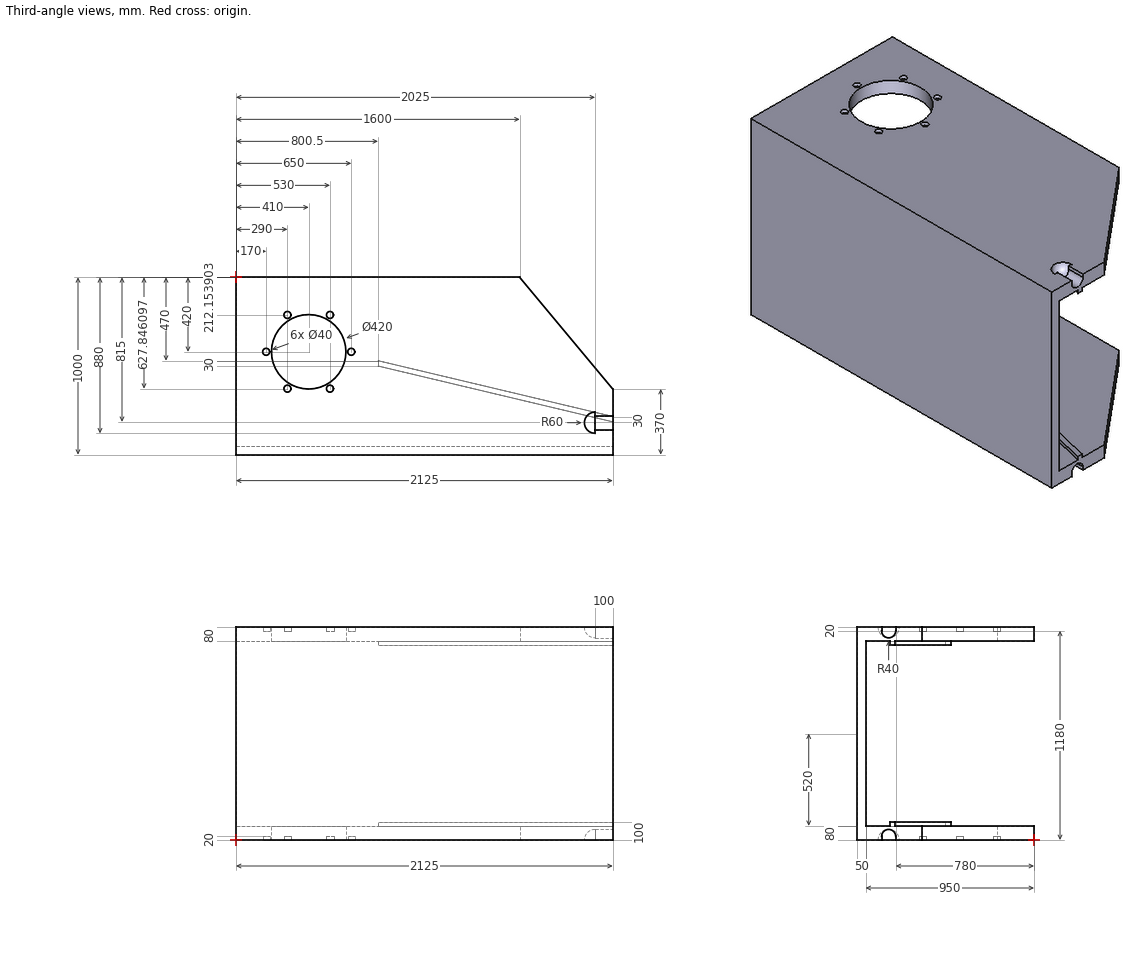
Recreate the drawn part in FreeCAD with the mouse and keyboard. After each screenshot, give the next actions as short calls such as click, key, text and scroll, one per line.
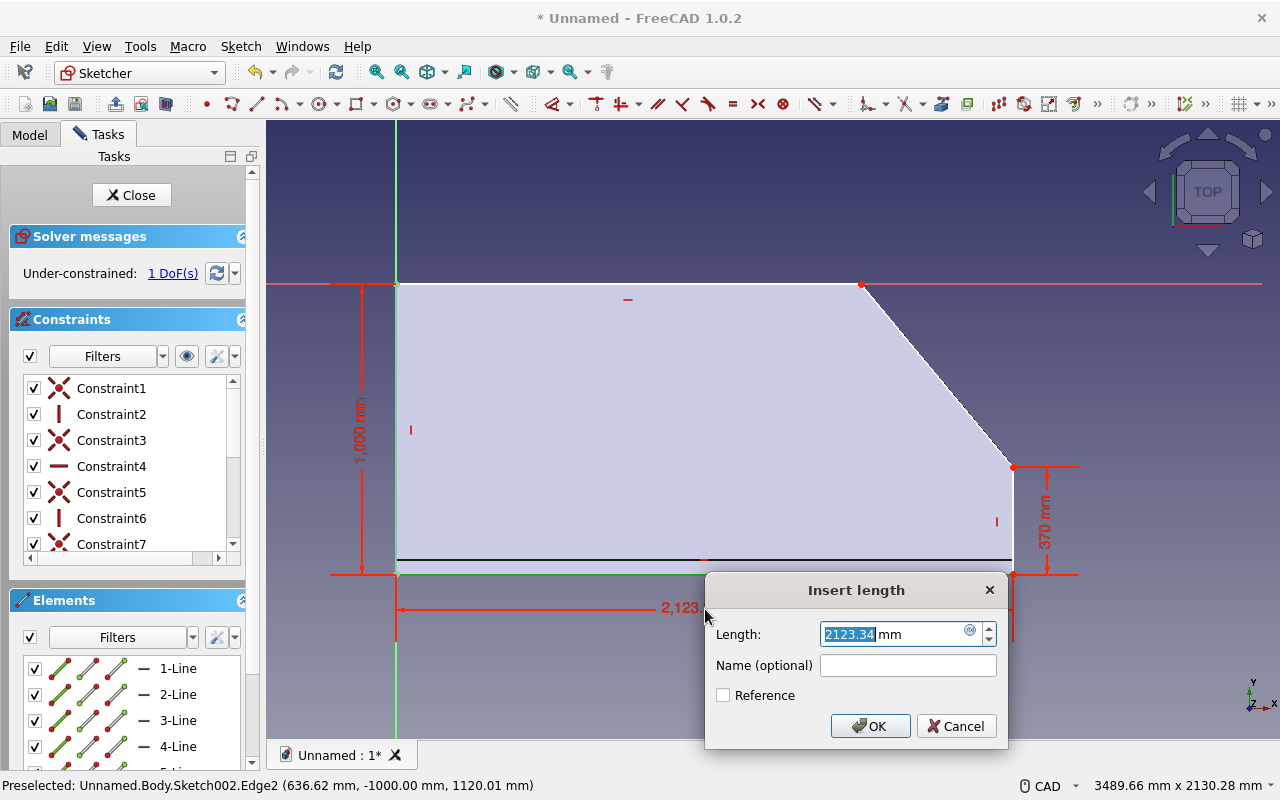
text(2125)
key(Return)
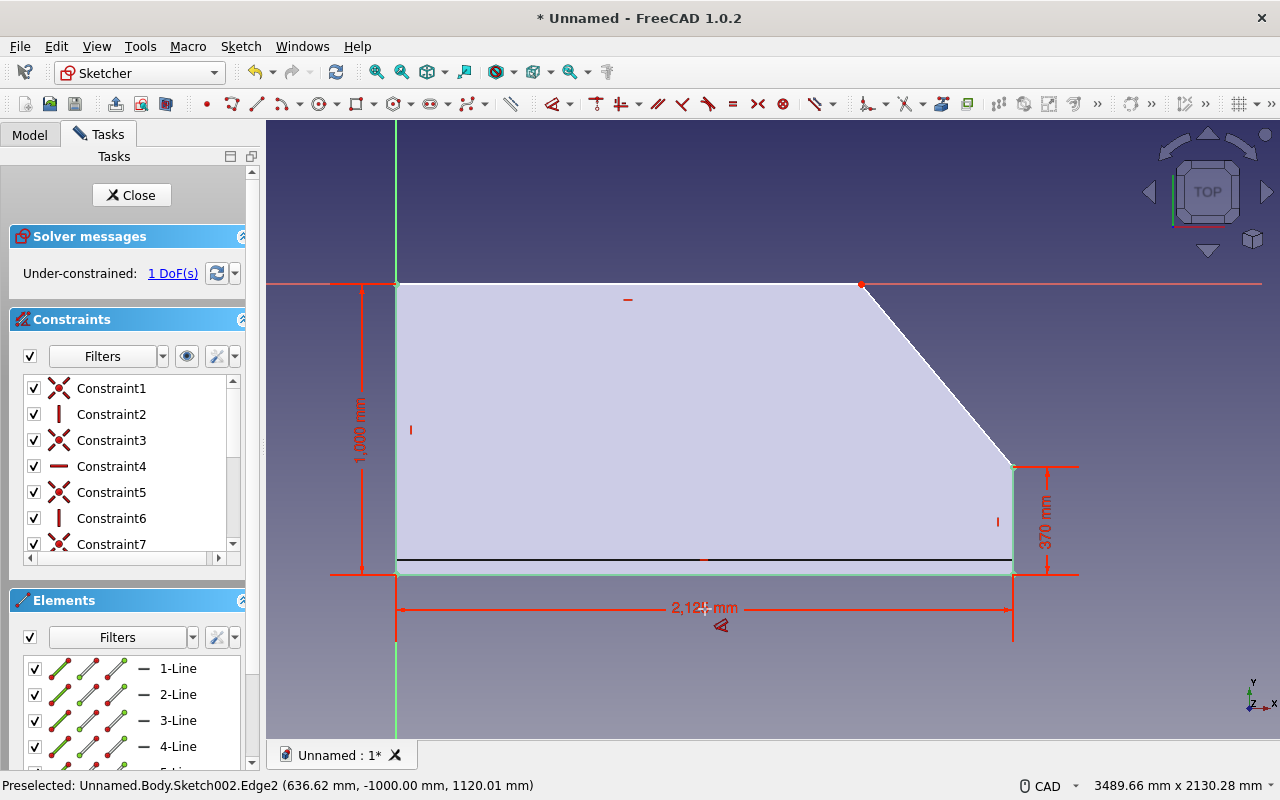
click(722, 284)
click(629, 250)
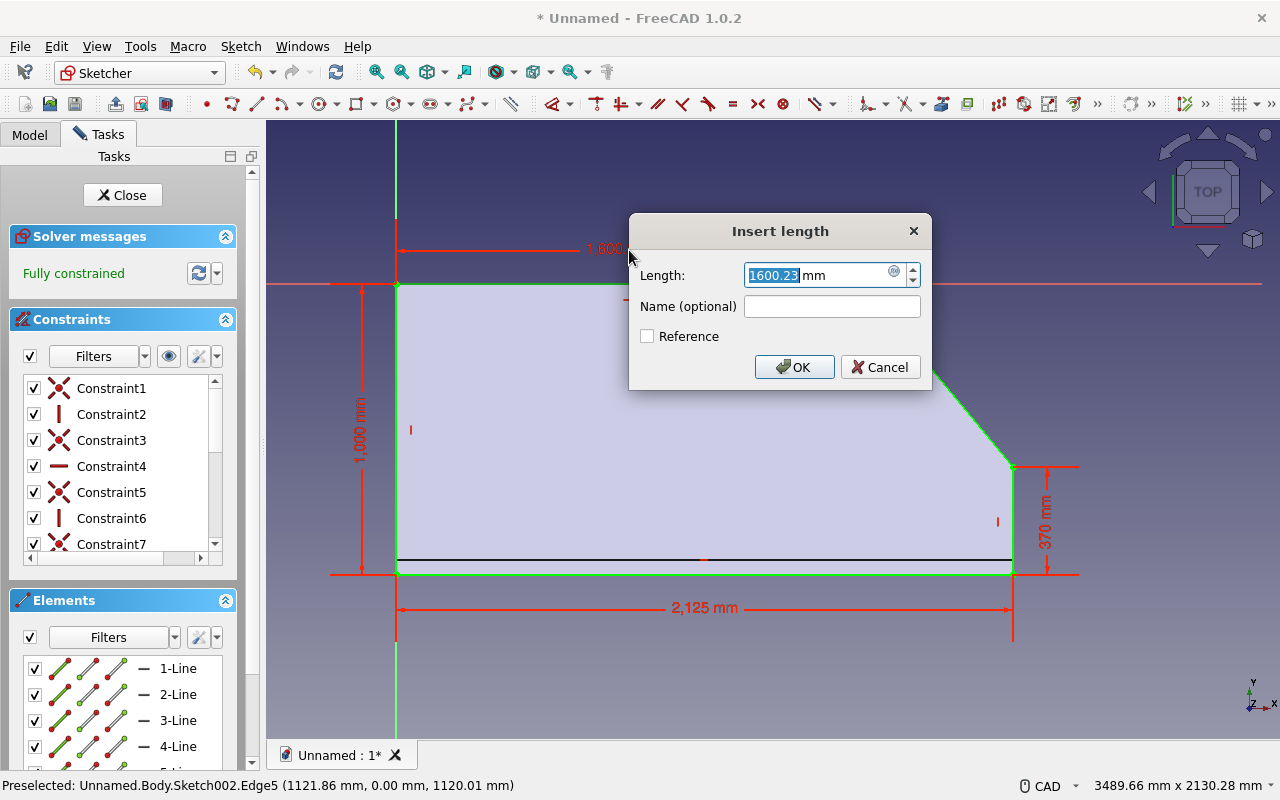
text(1600)
key(Return)
key(Escape)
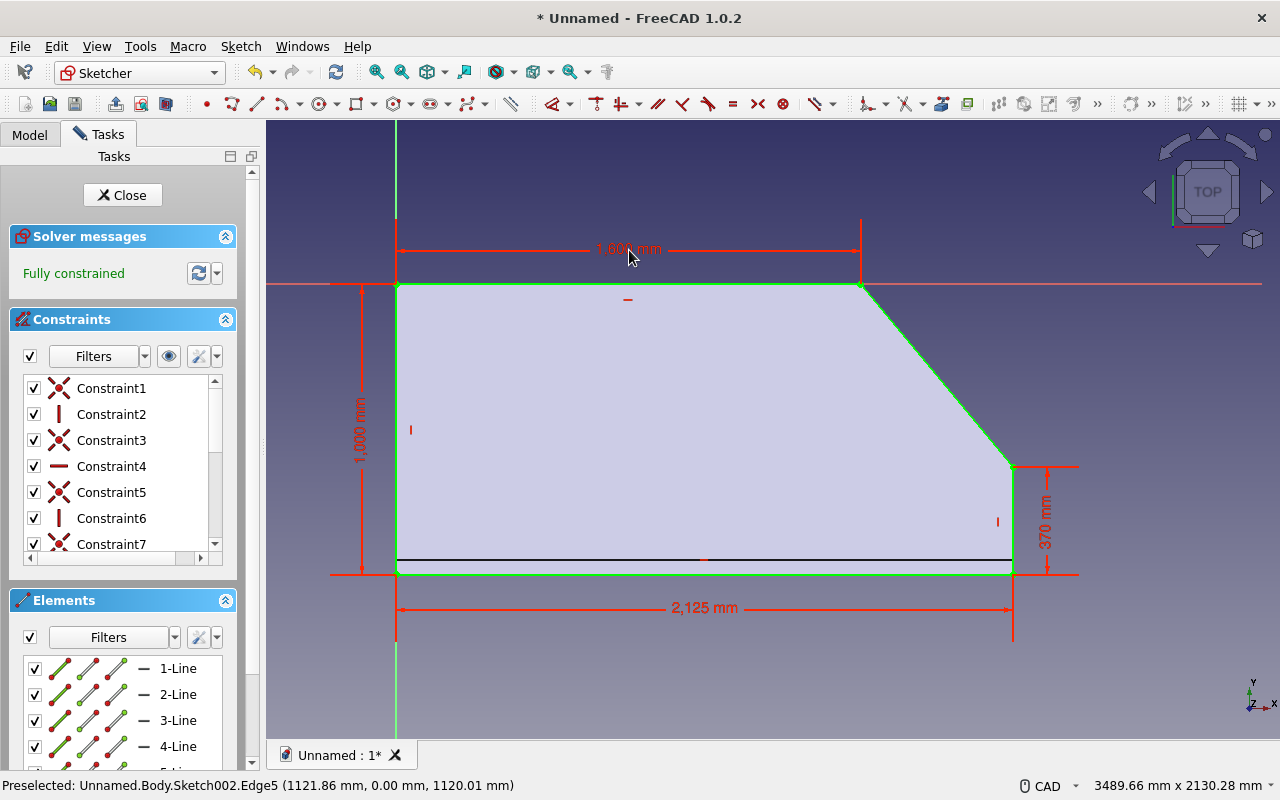
click(123, 195)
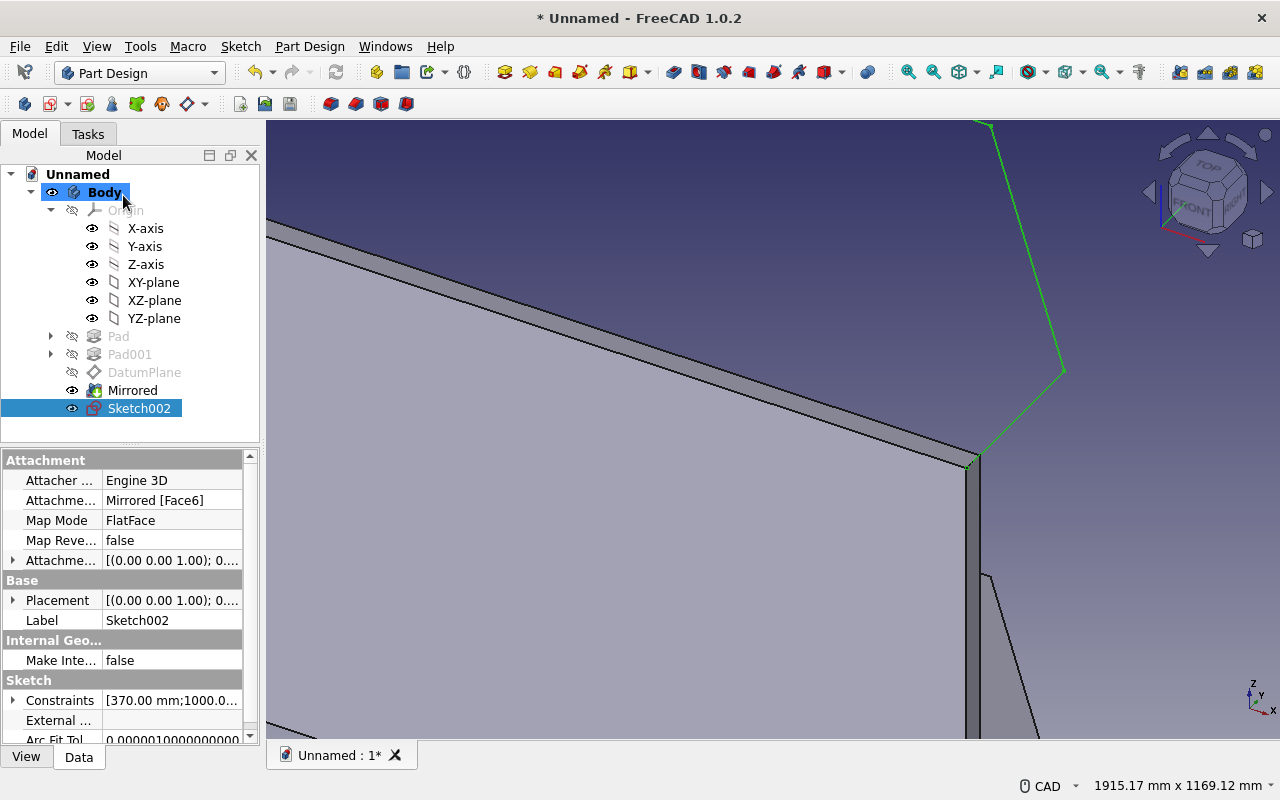
click(505, 72)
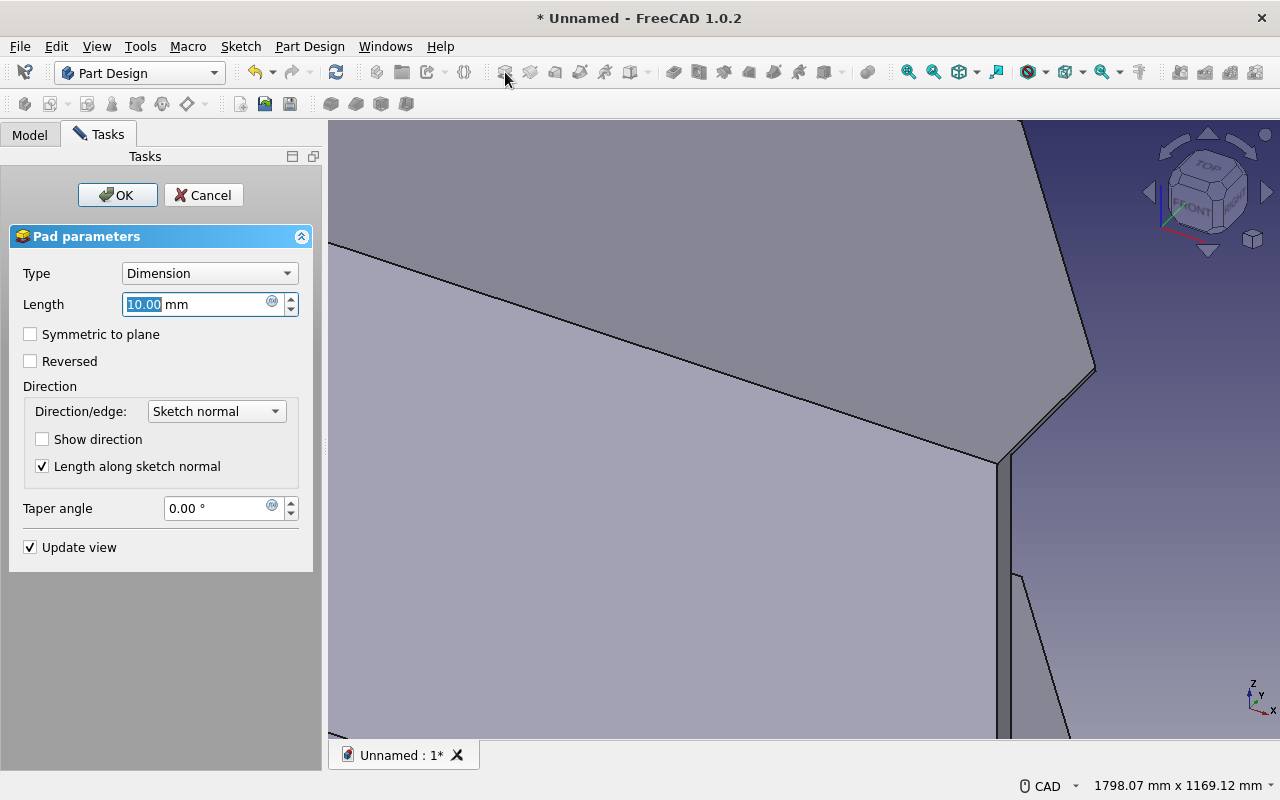
text(80)
key(Tab)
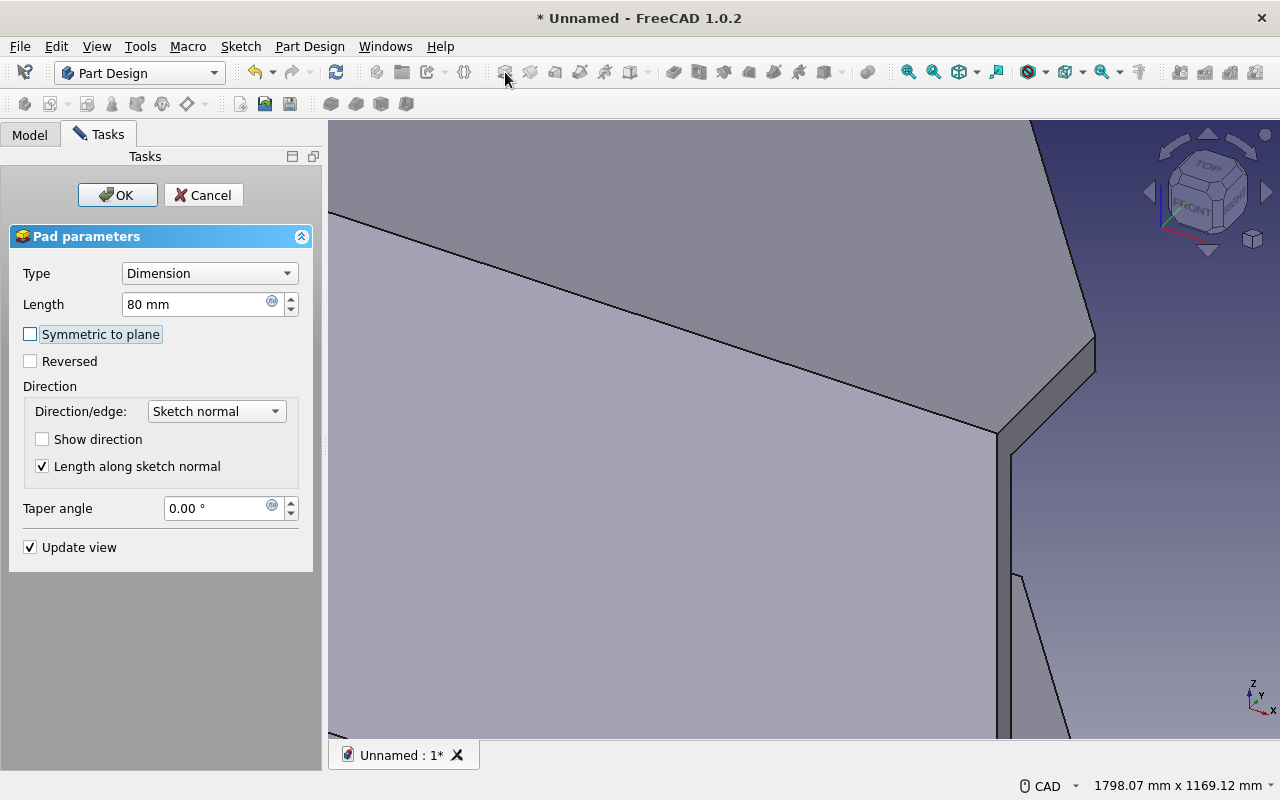
click(118, 195)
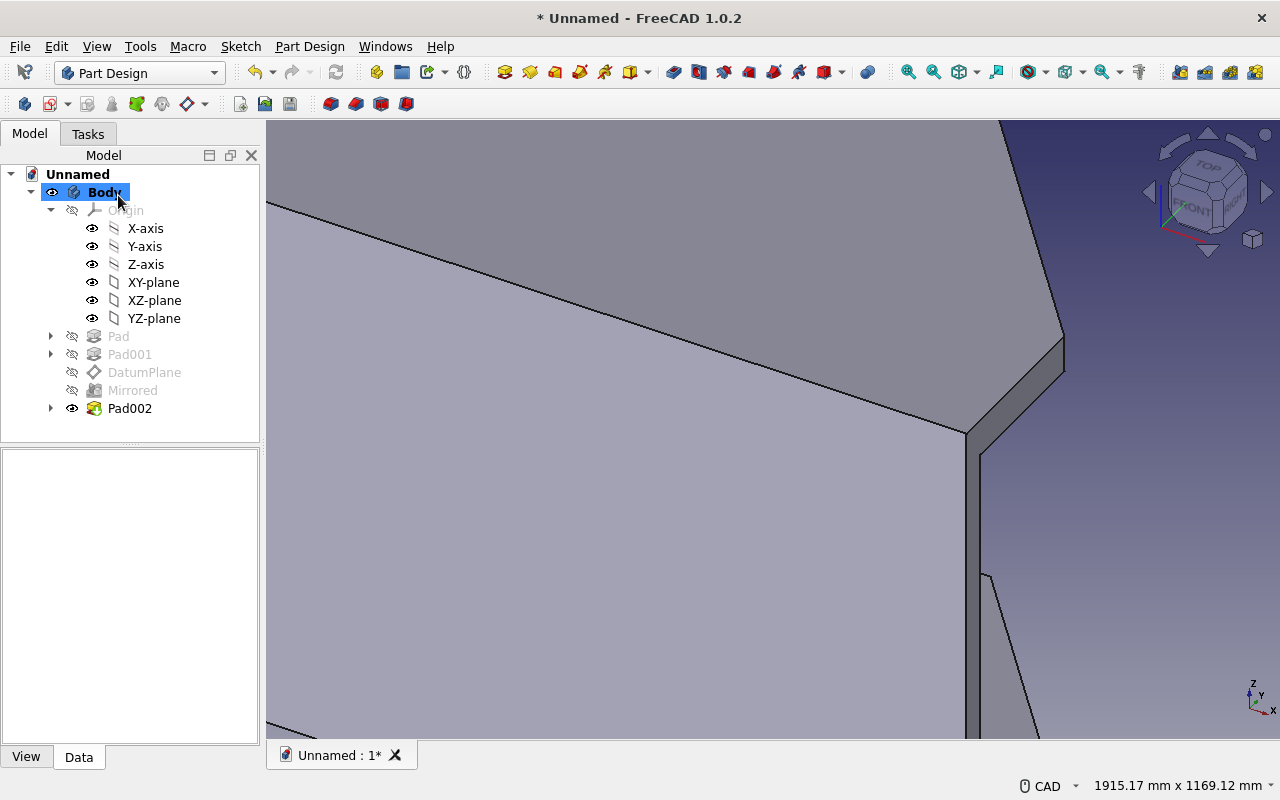
key(v)
key(f)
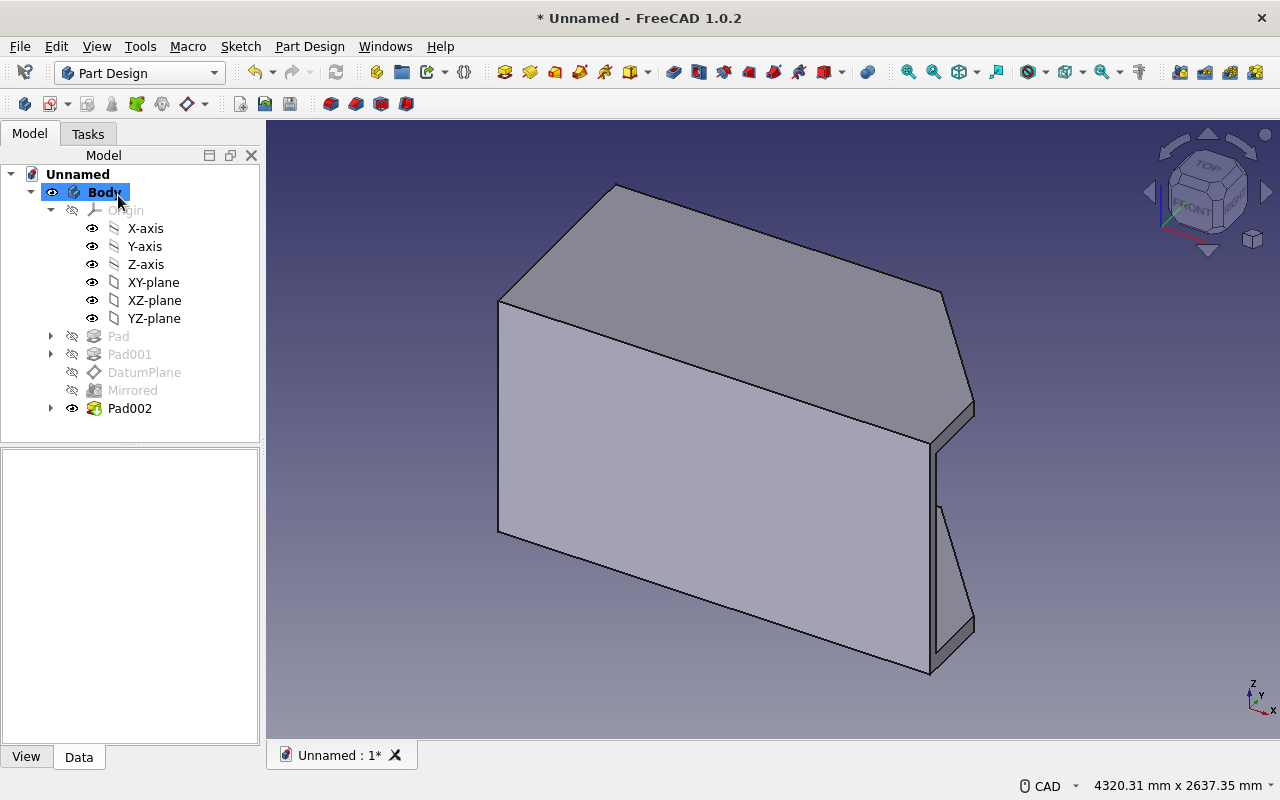
click(50, 104)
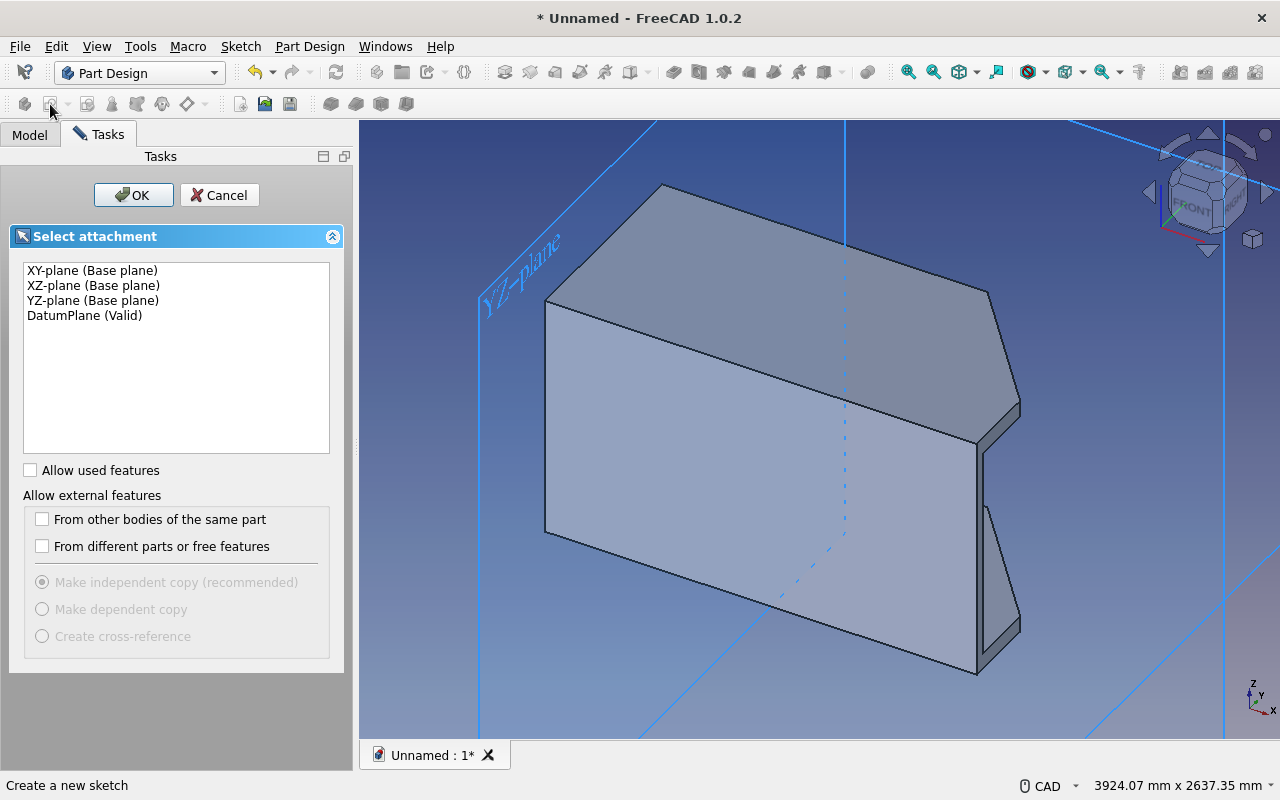
click(84, 270)